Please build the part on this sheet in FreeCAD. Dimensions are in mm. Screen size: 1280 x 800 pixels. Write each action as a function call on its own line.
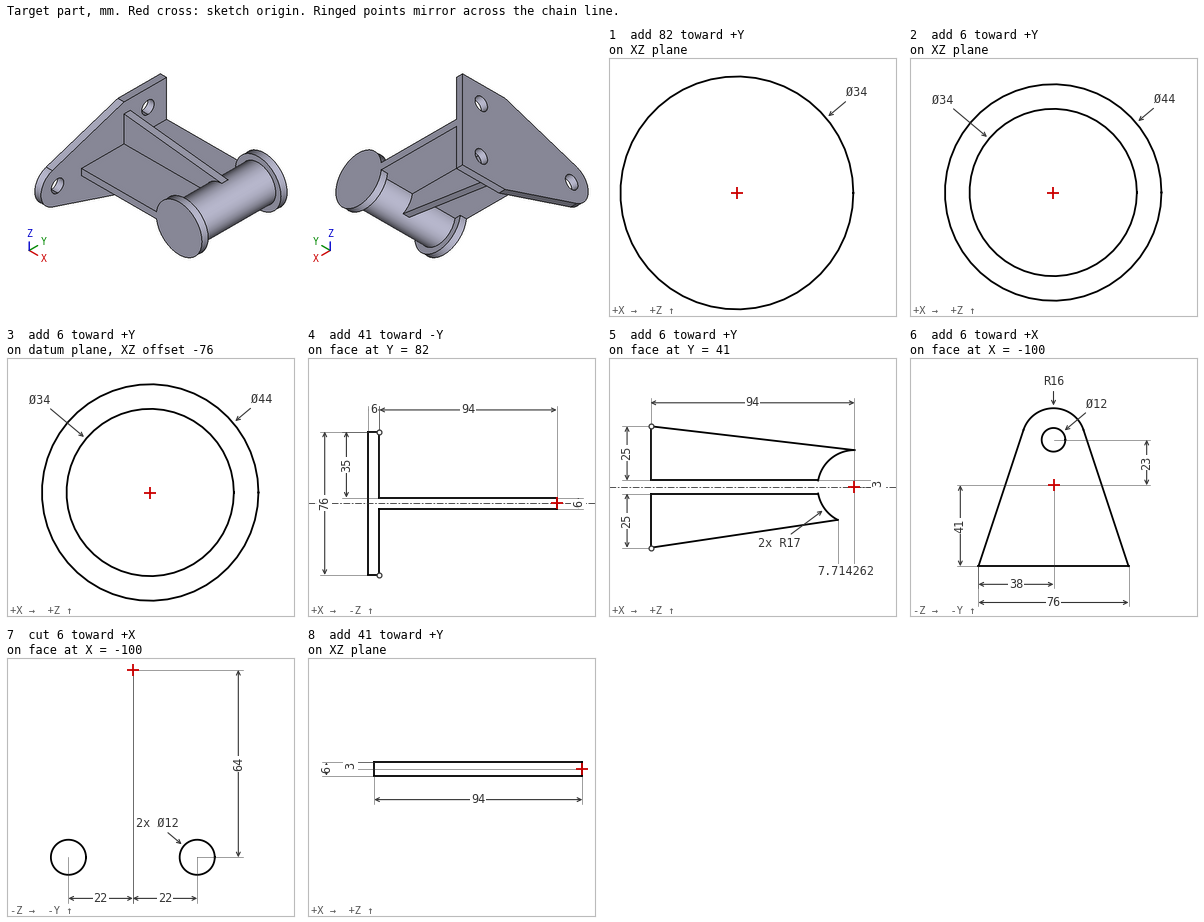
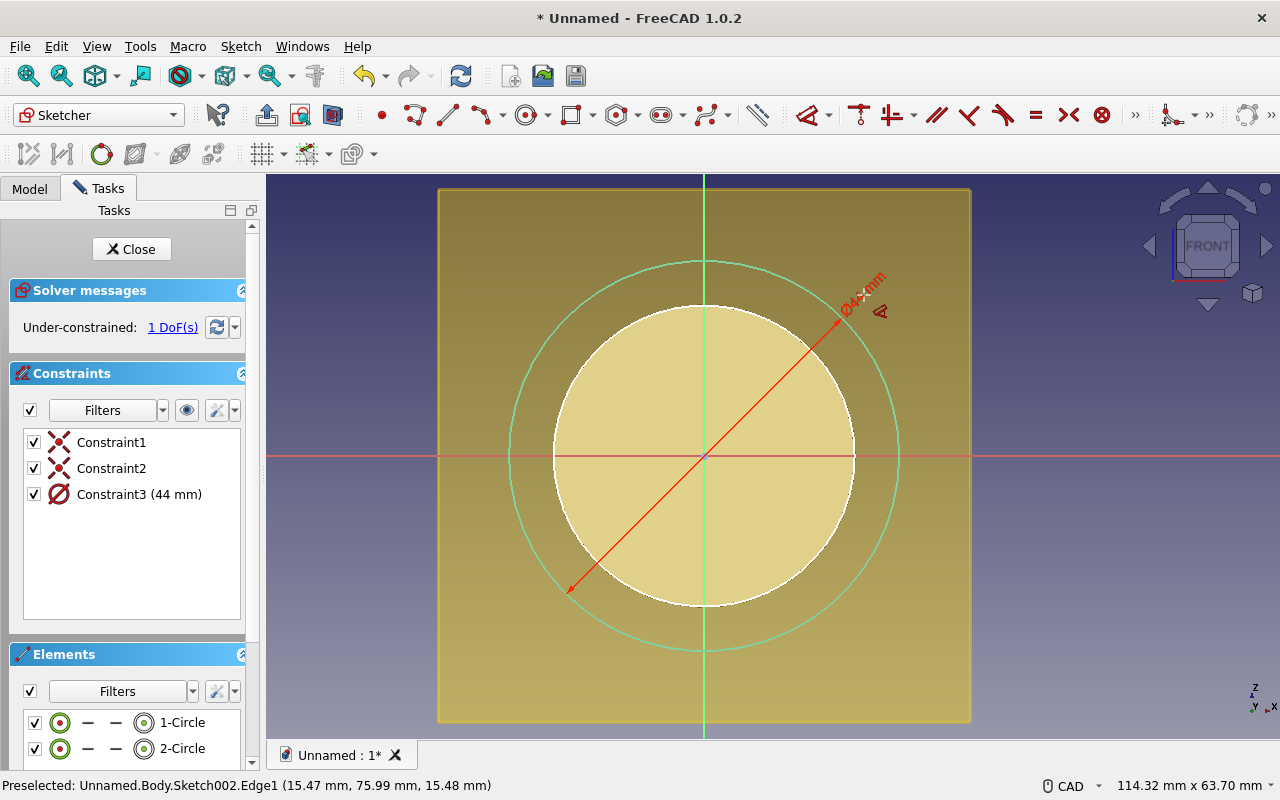
click(810, 349)
click(925, 390)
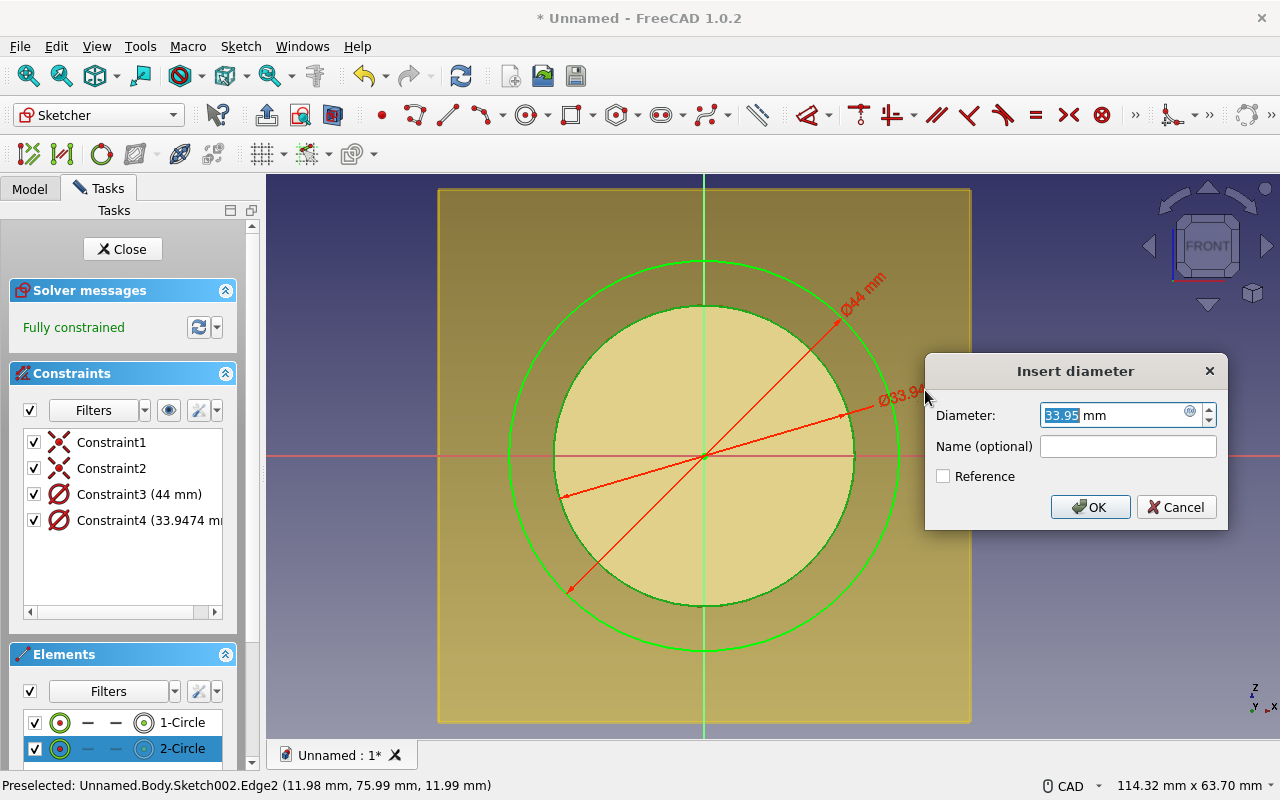
text(34)
key(Return)
key(Escape)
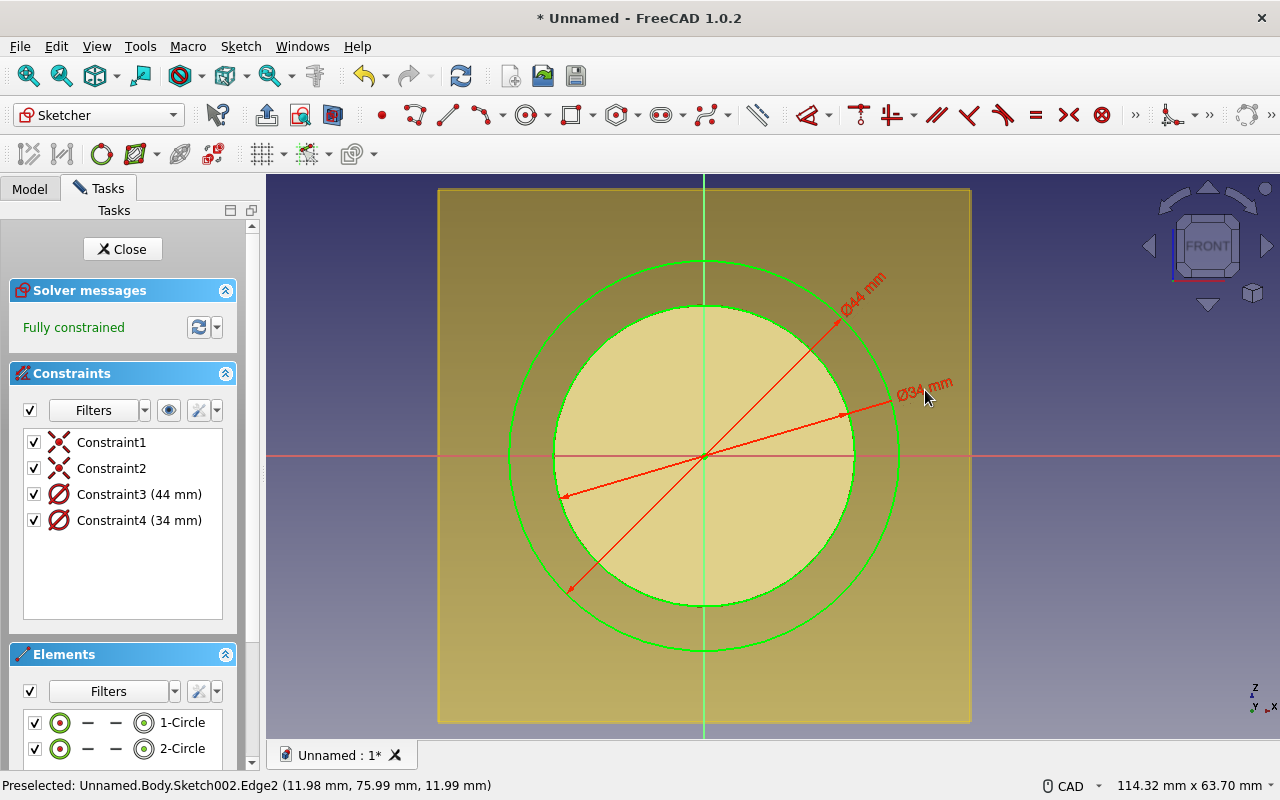
click(123, 249)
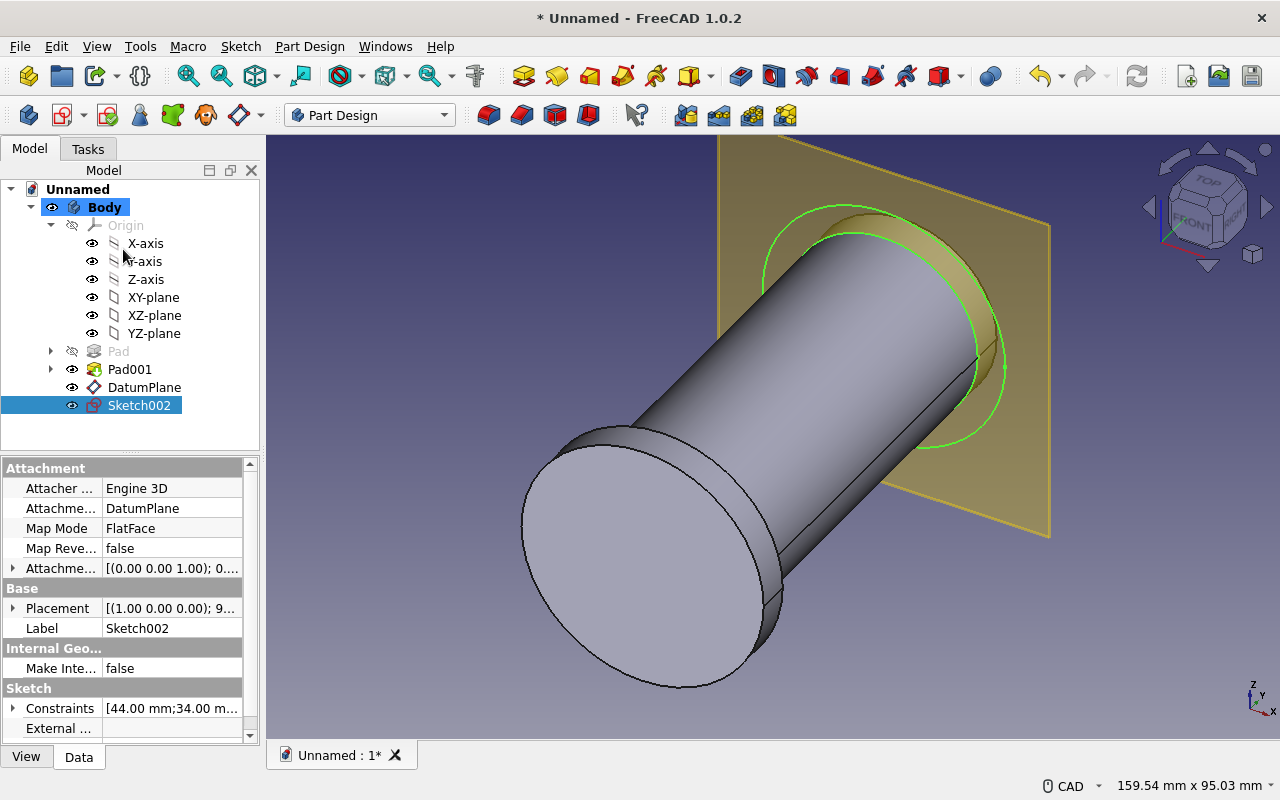
click(524, 76)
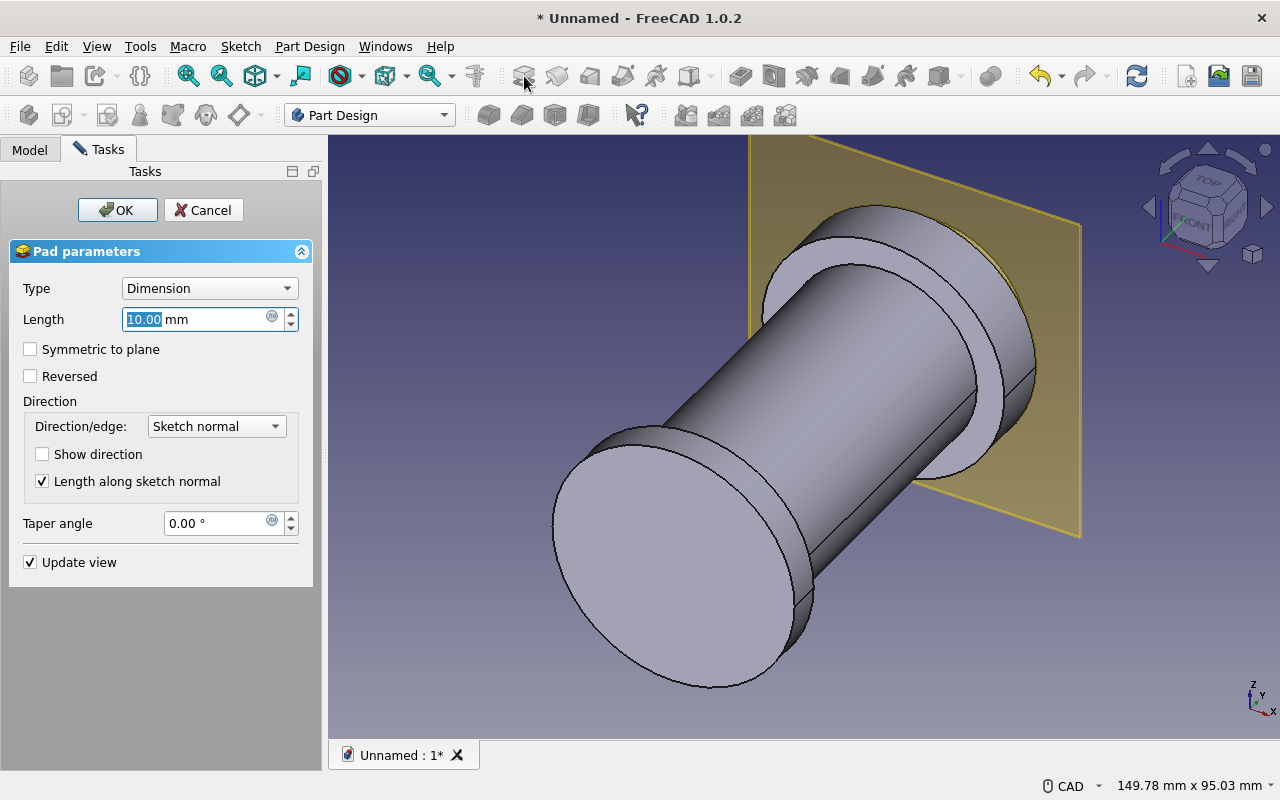
text(6)
key(Tab)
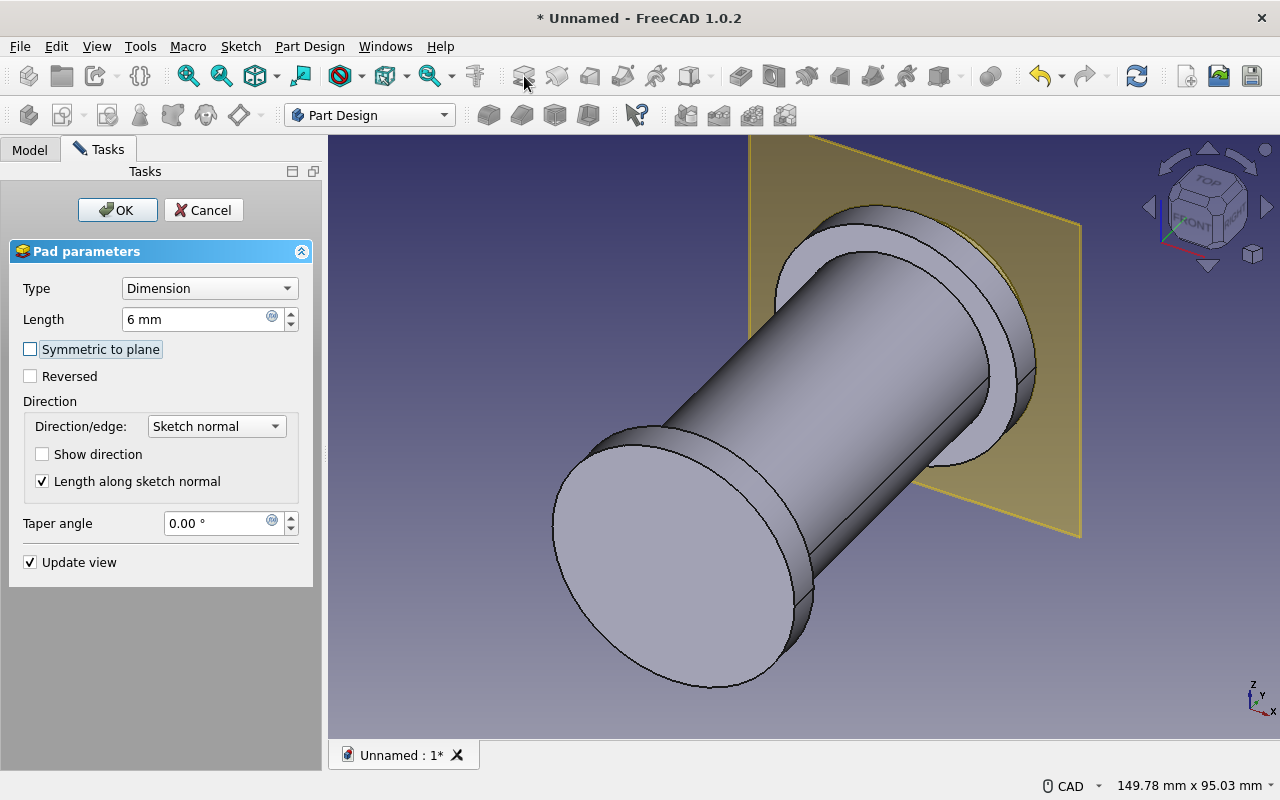
click(31, 376)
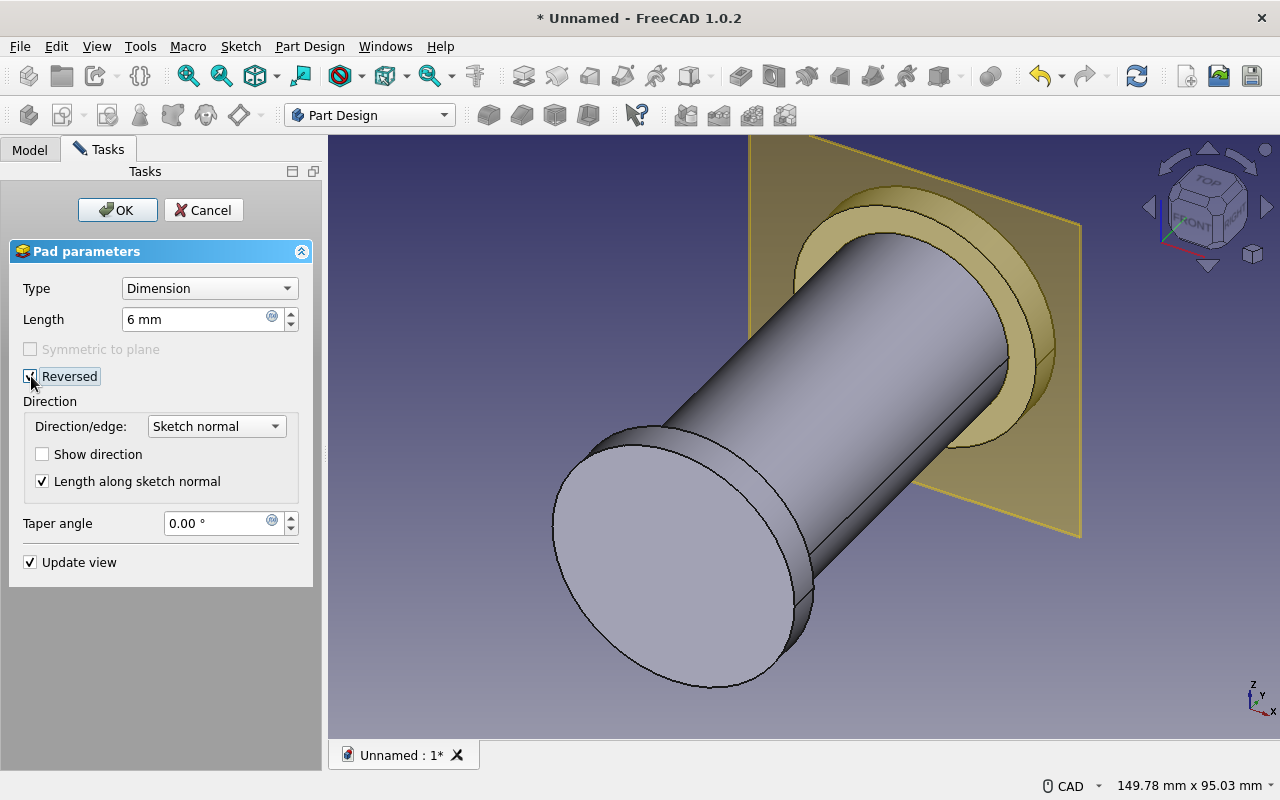
click(118, 210)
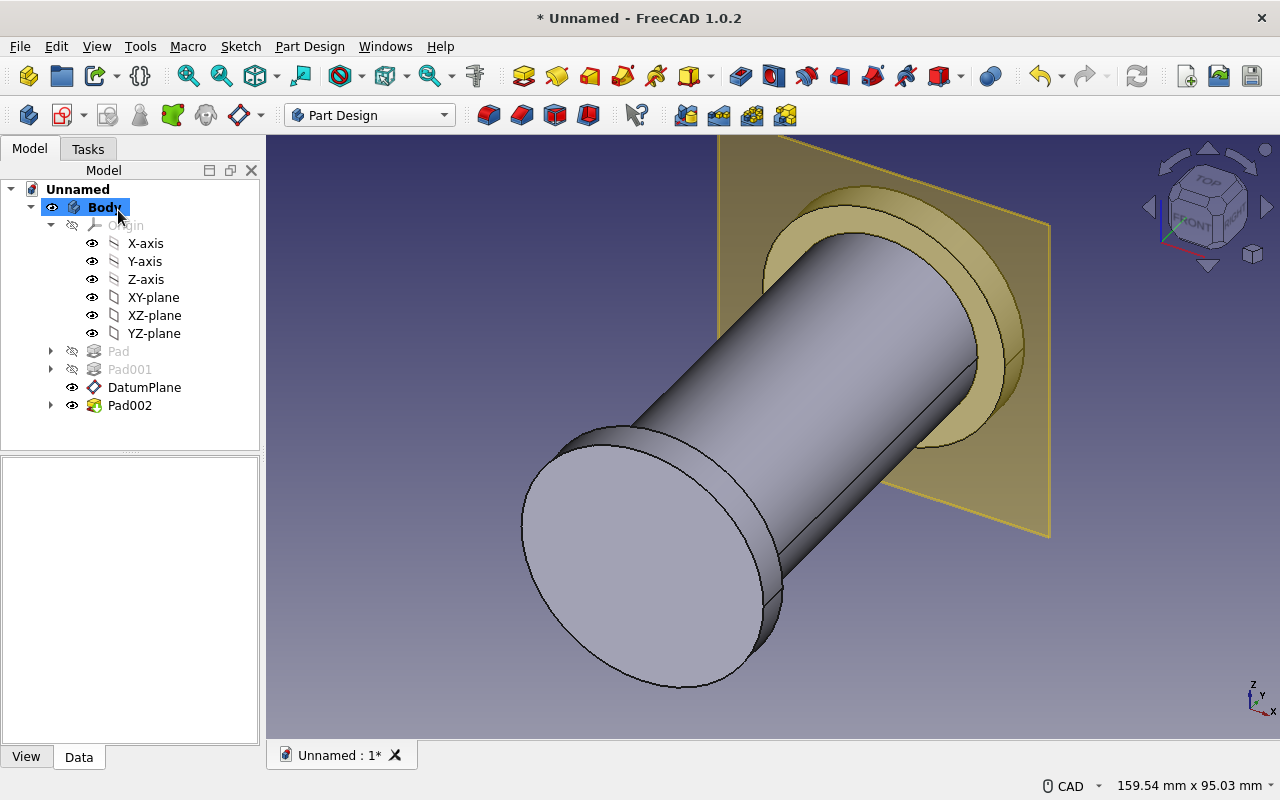
click(117, 387)
key(space)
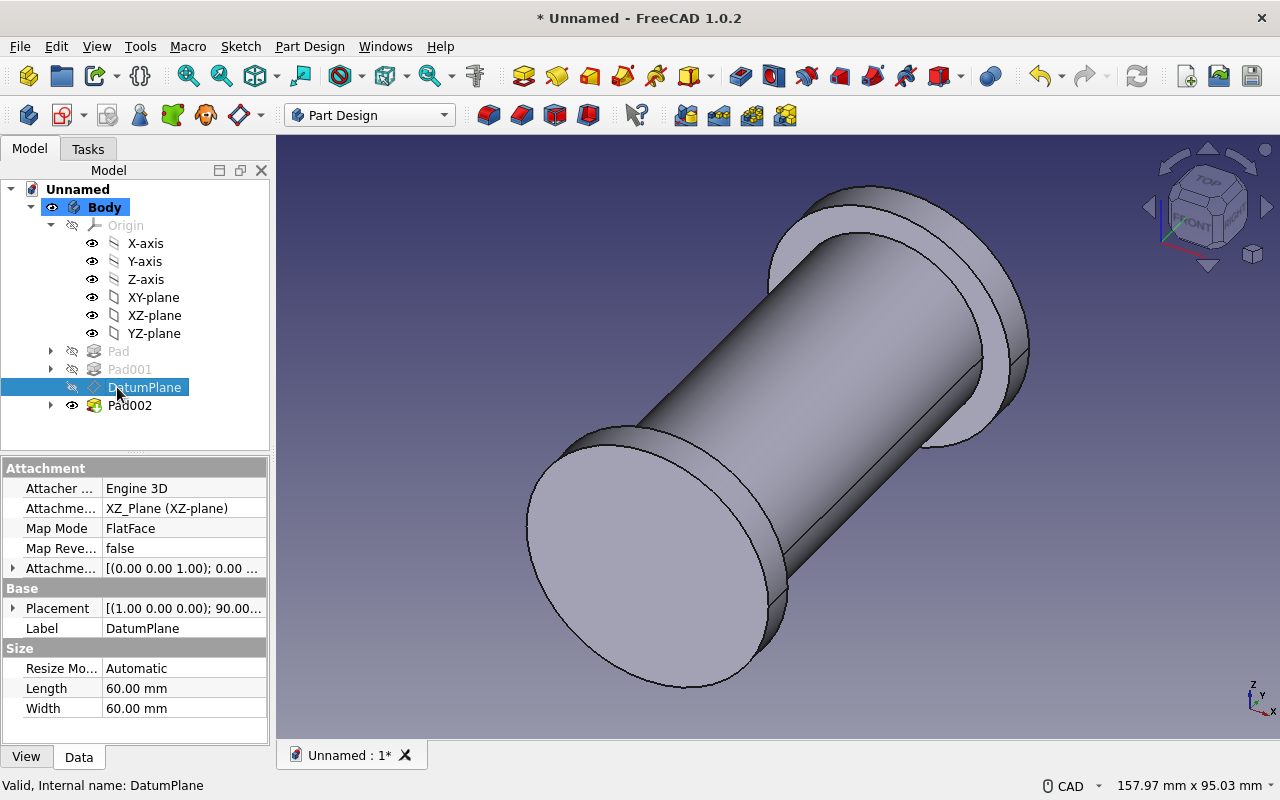
key(4)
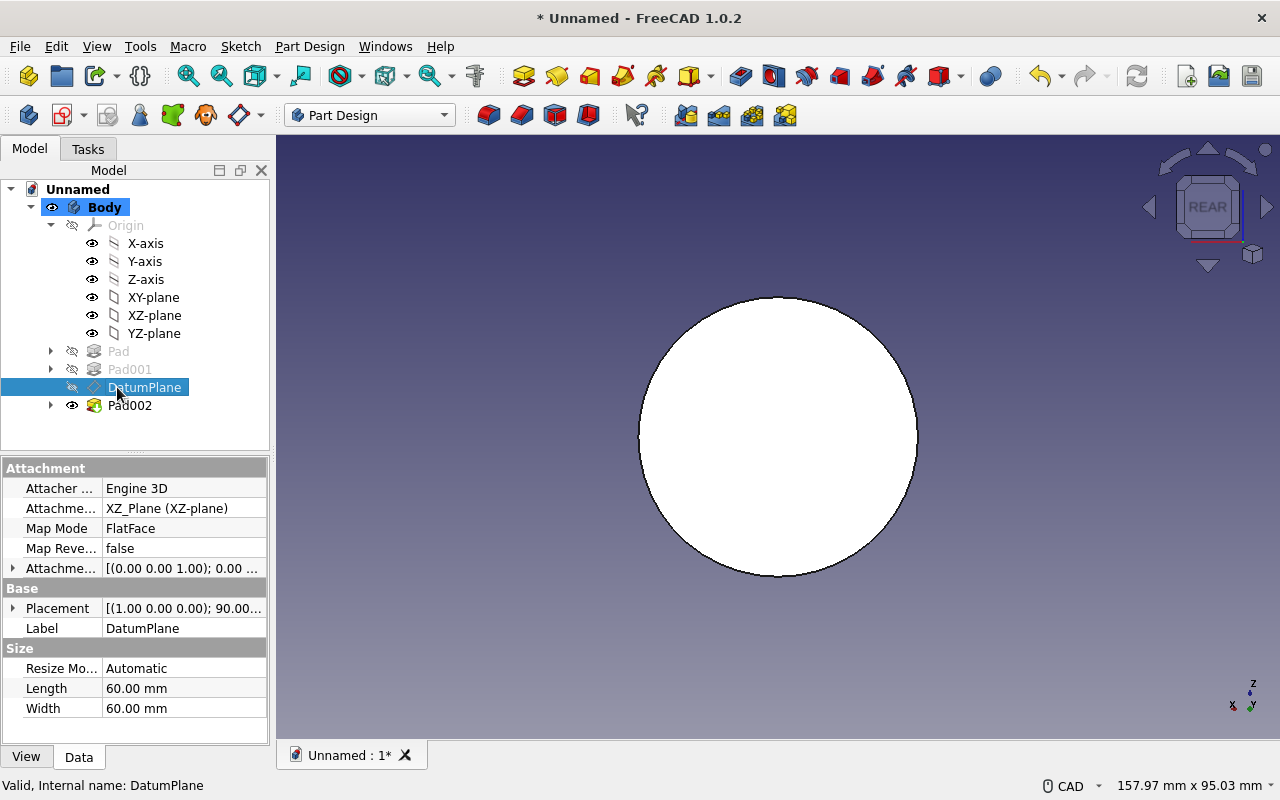
click(778, 436)